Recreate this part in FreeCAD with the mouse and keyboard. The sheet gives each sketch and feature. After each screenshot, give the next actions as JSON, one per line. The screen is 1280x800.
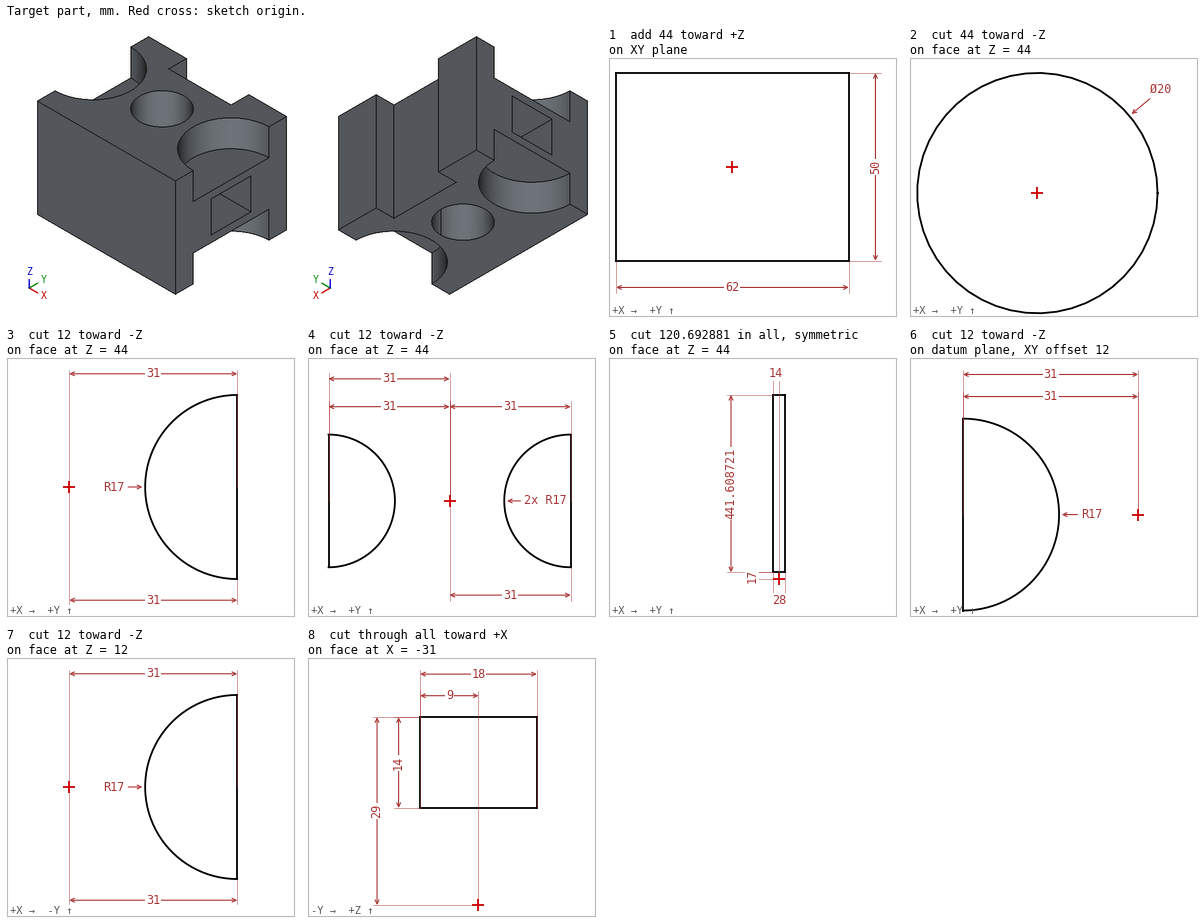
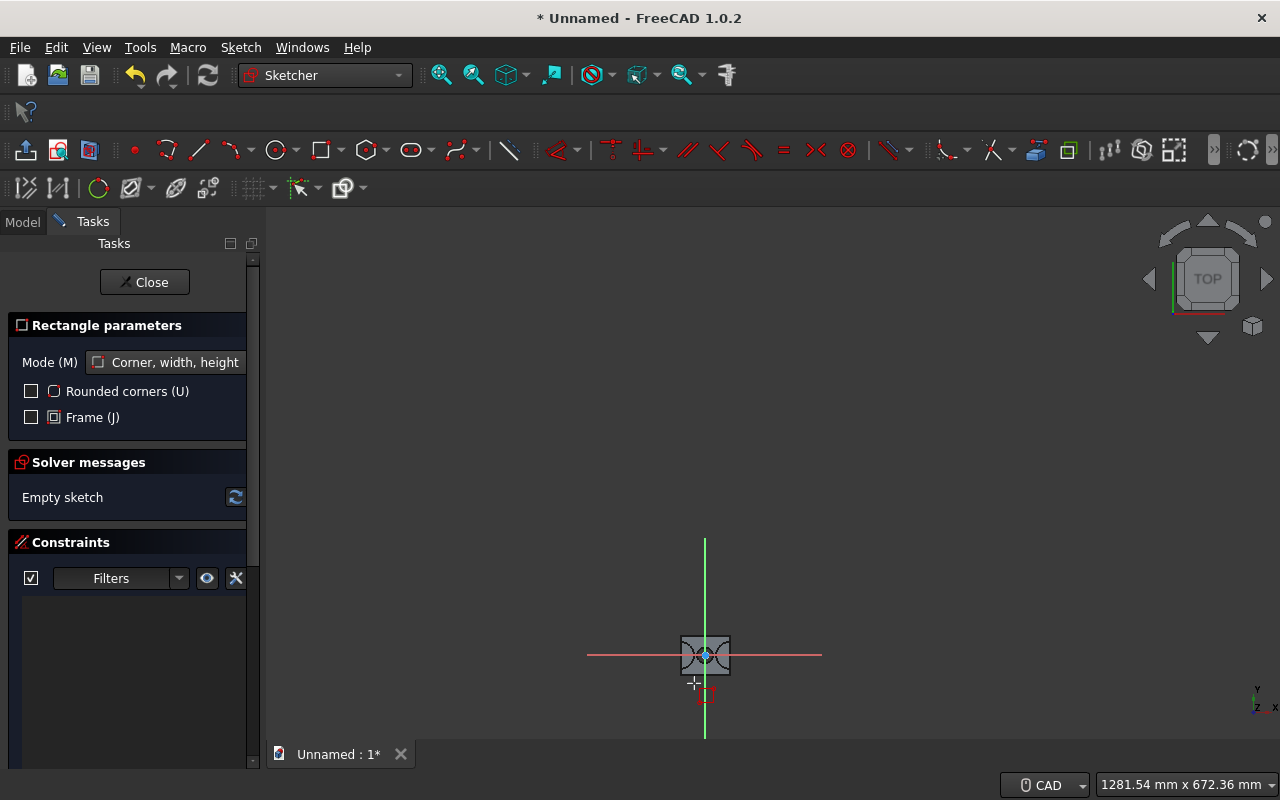
{"action": "scroll", "coordinate": [694, 292], "scroll_direction": "up", "scroll_amount": 2}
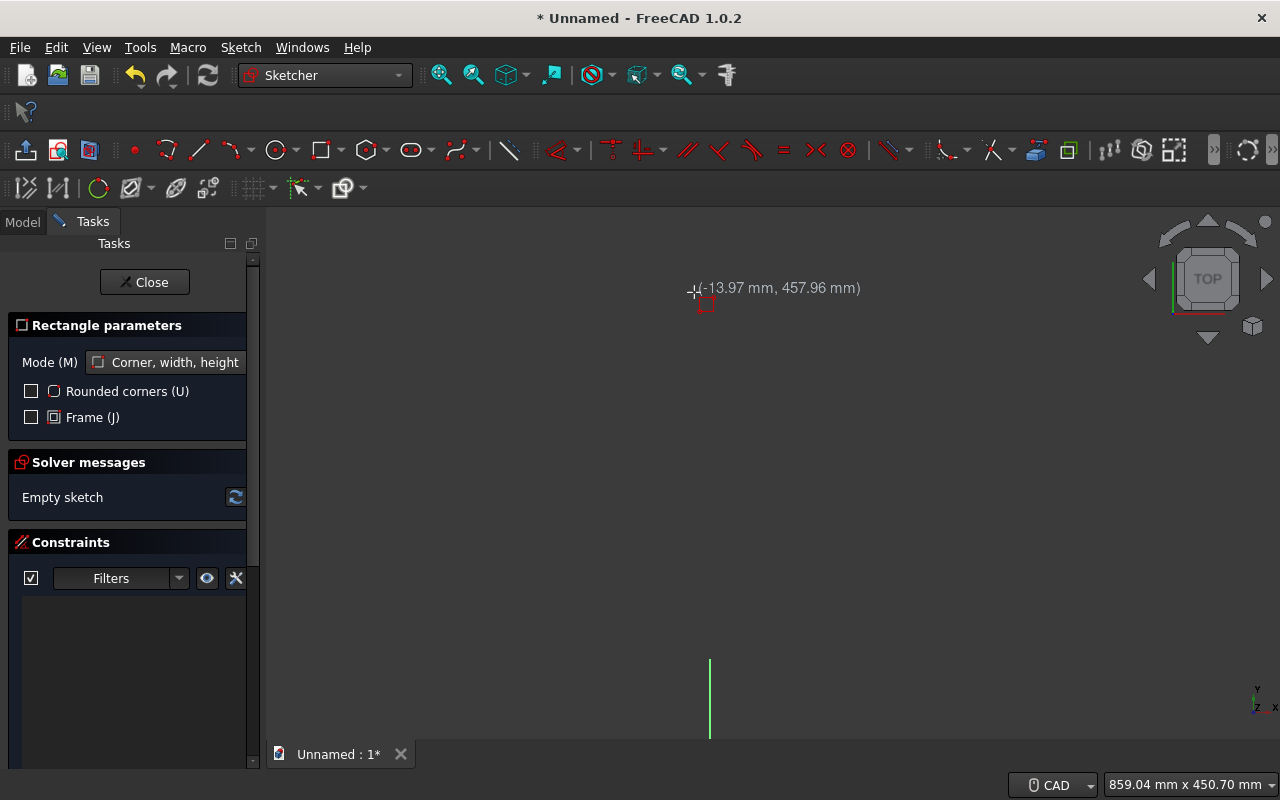
{"action": "left_click", "coordinate": [694, 293]}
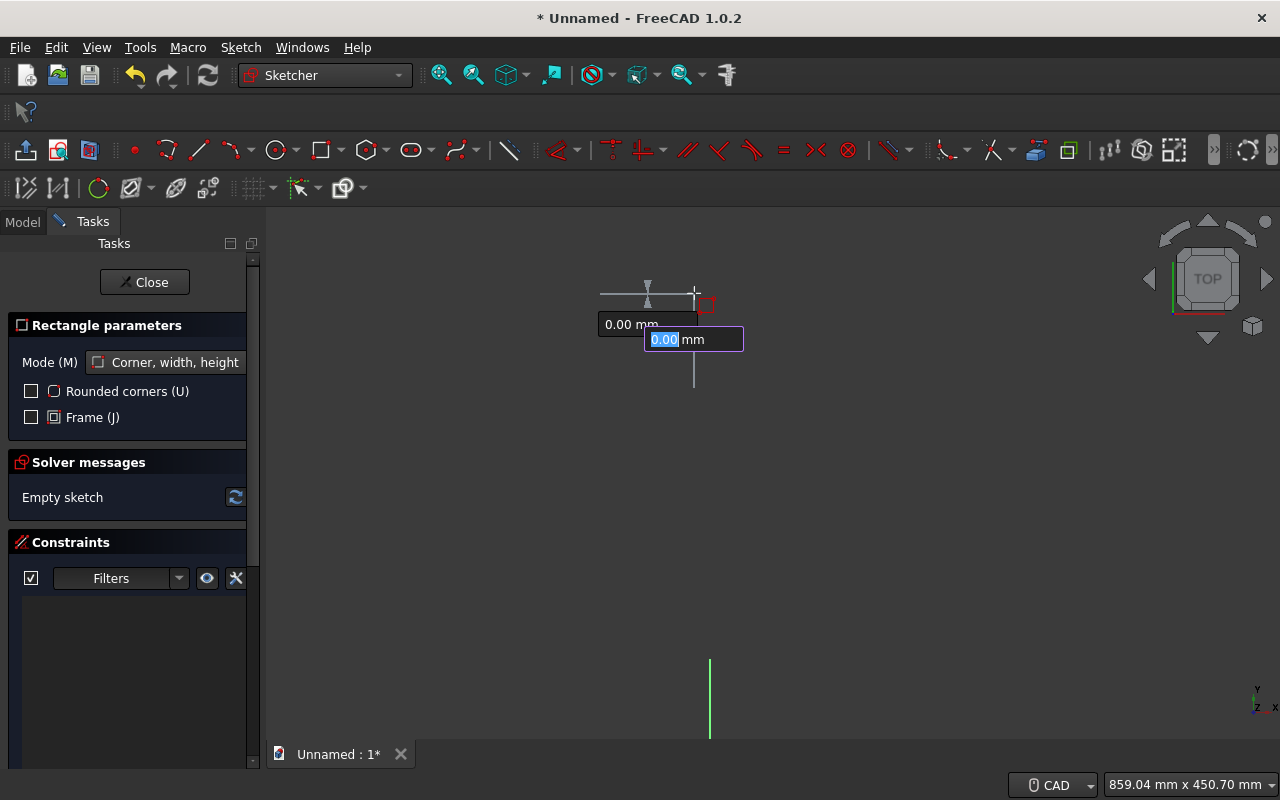
{"action": "scroll", "coordinate": [693, 289], "scroll_direction": "down", "scroll_amount": 2}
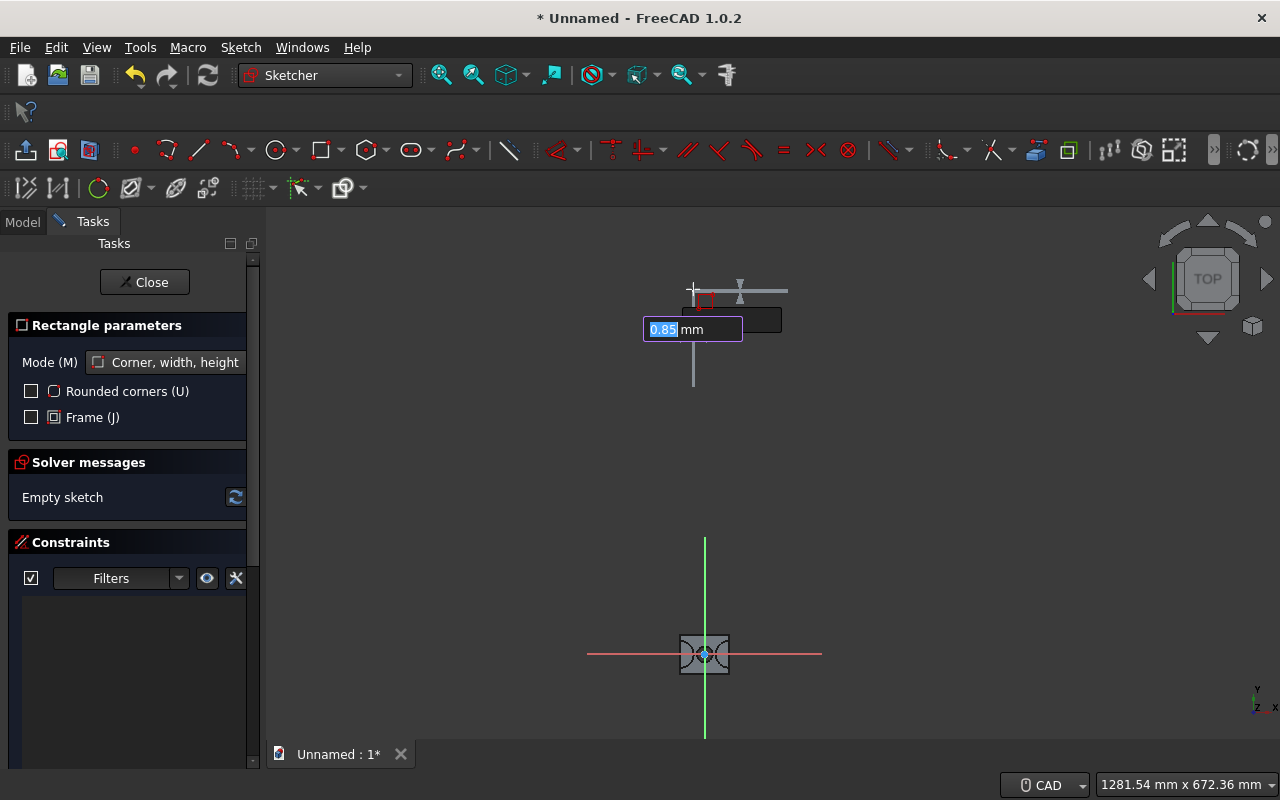
{"action": "scroll", "coordinate": [716, 641], "scroll_direction": "up", "scroll_amount": 2}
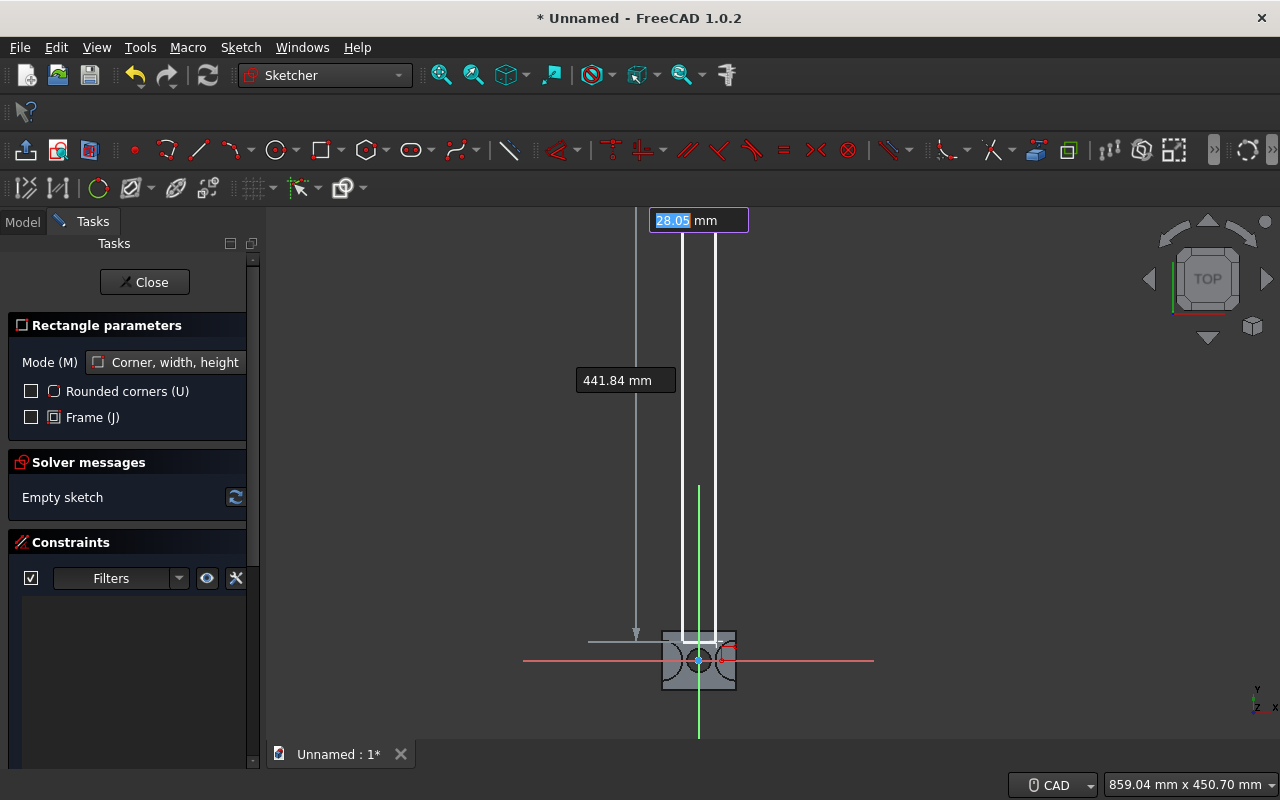
{"action": "left_click", "coordinate": [715, 640]}
{"action": "key", "text": "Escape"}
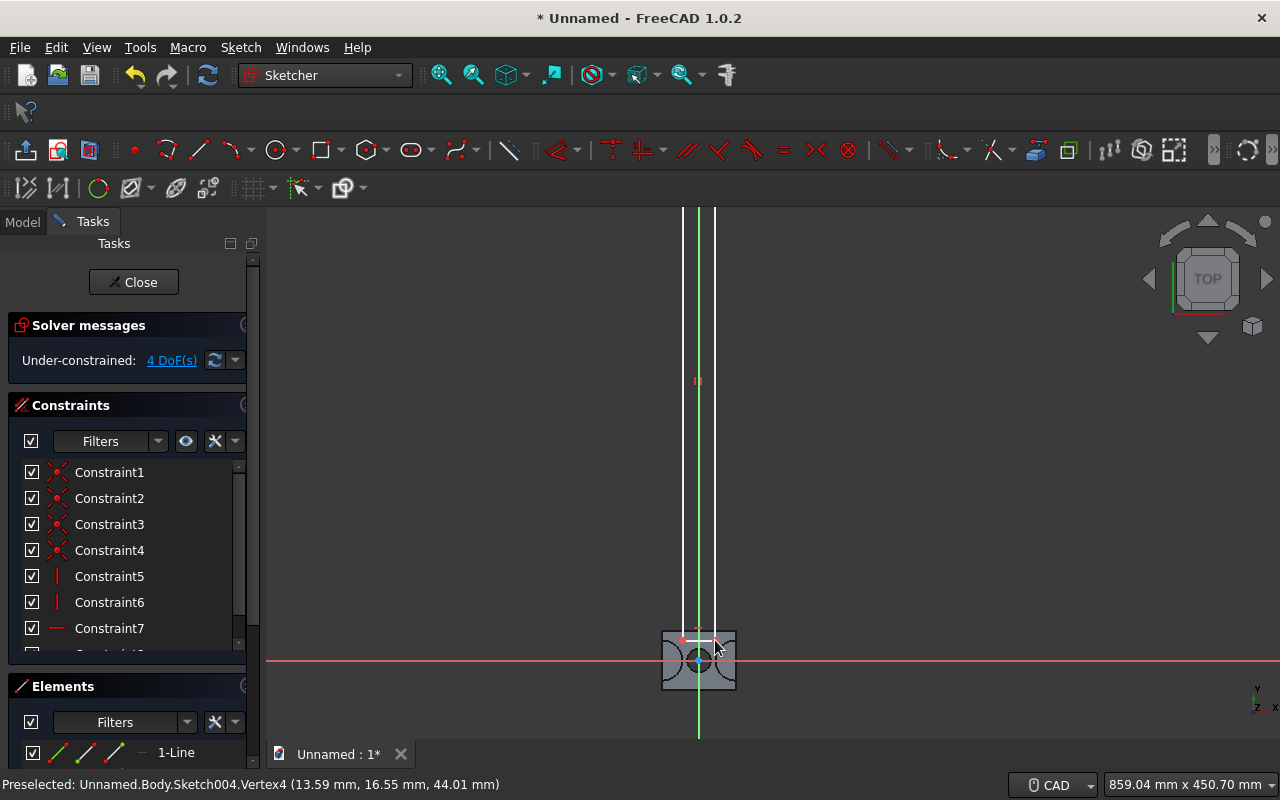
{"action": "key", "text": "d"}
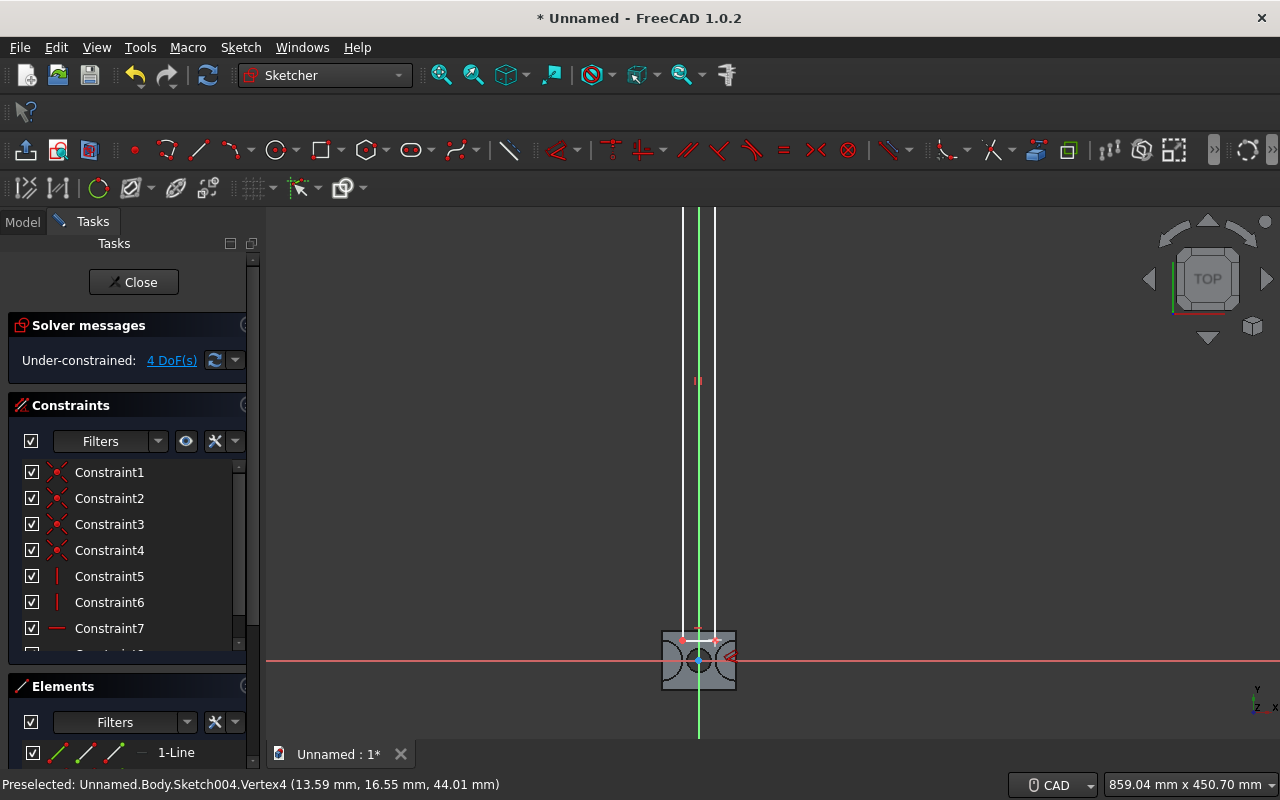
{"action": "left_click", "coordinate": [696, 641]}
{"action": "left_click", "coordinate": [691, 675]}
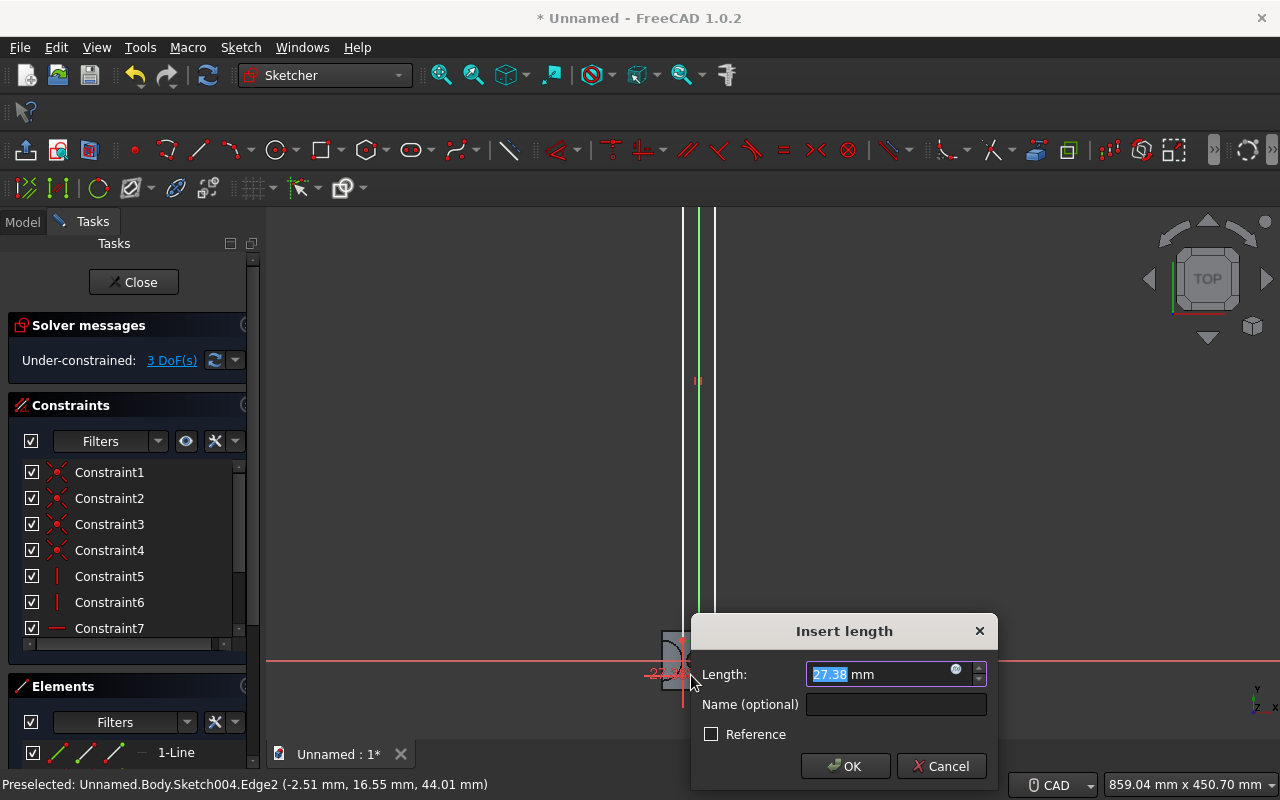
{"action": "type", "text": "28"}
{"action": "key", "text": "Return"}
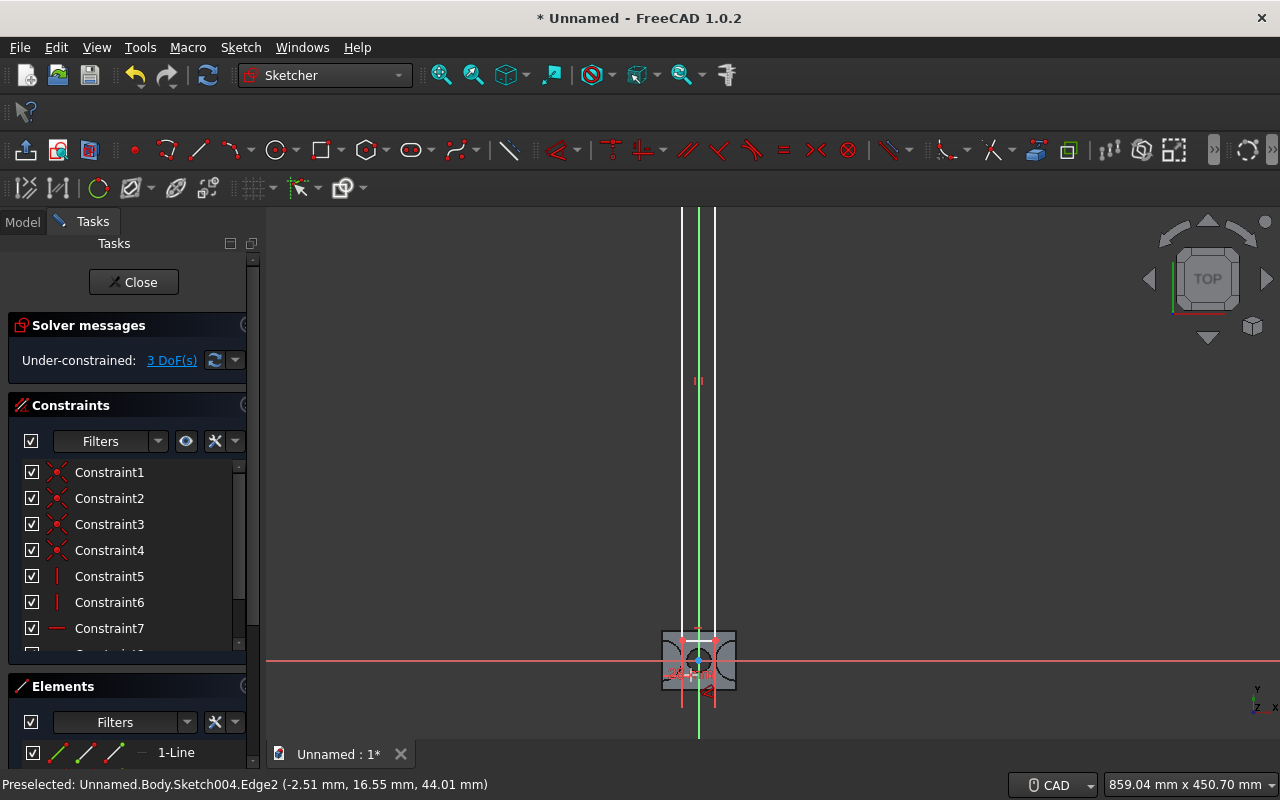
{"action": "scroll", "coordinate": [716, 642], "scroll_direction": "down", "scroll_amount": 2}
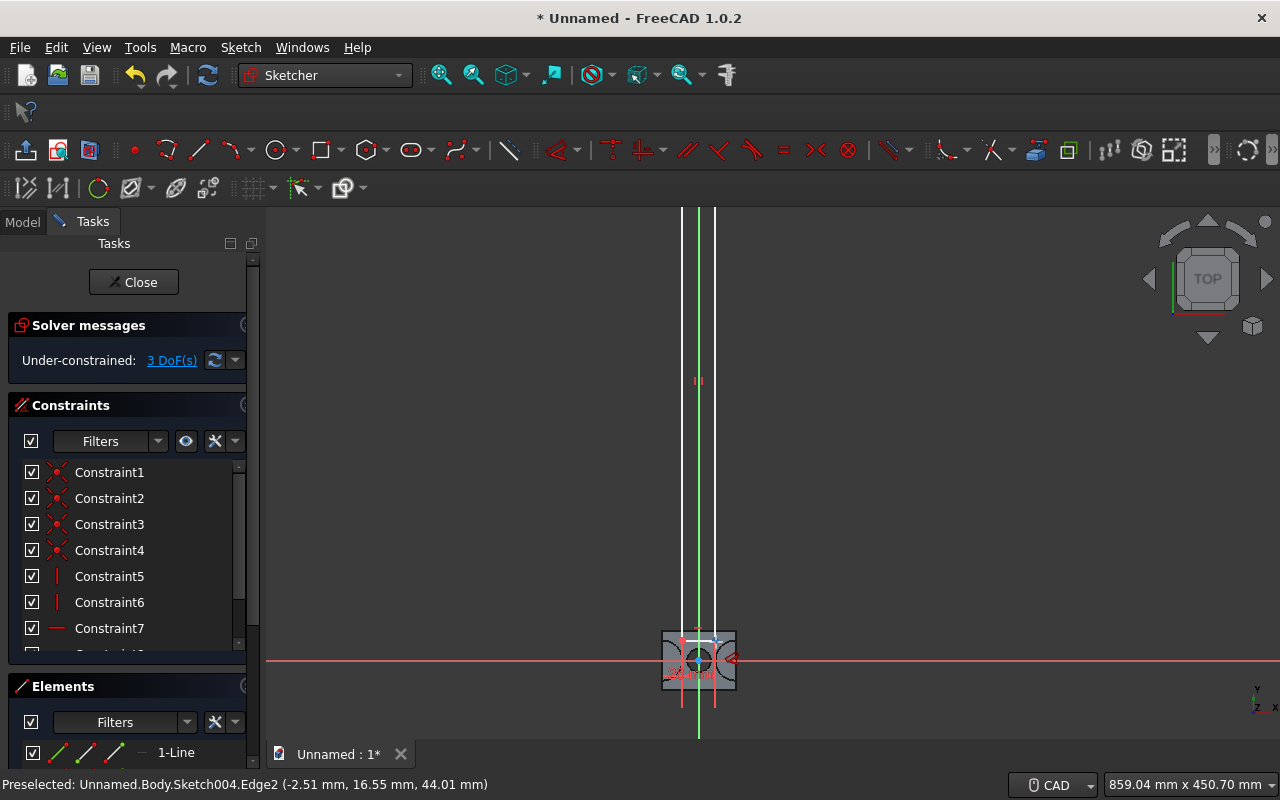
{"action": "scroll", "coordinate": [694, 293], "scroll_direction": "up", "scroll_amount": 7}